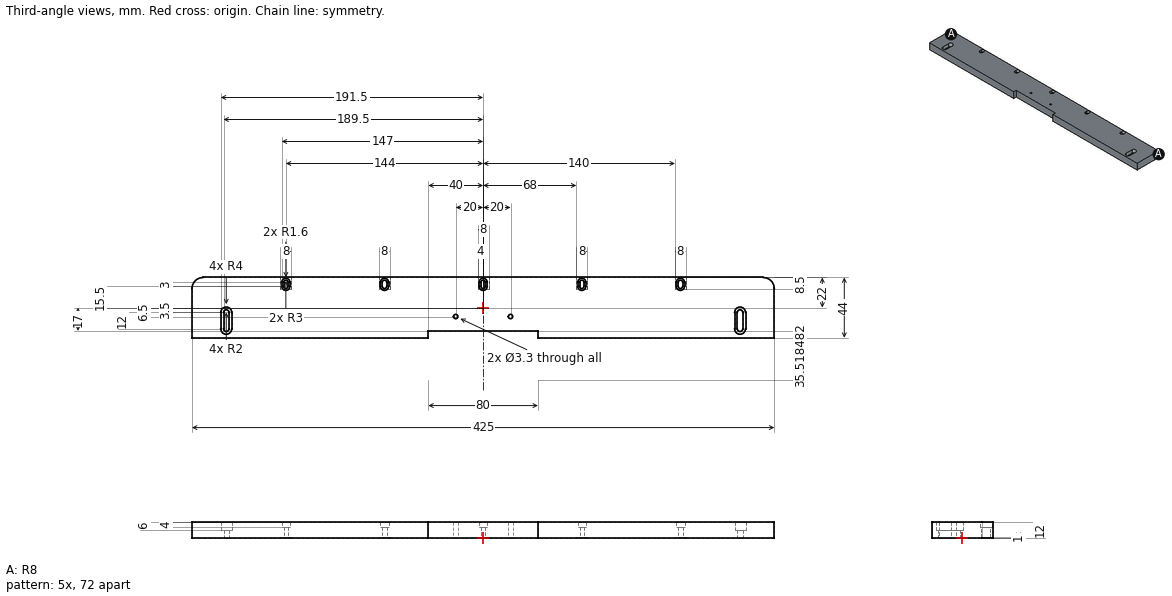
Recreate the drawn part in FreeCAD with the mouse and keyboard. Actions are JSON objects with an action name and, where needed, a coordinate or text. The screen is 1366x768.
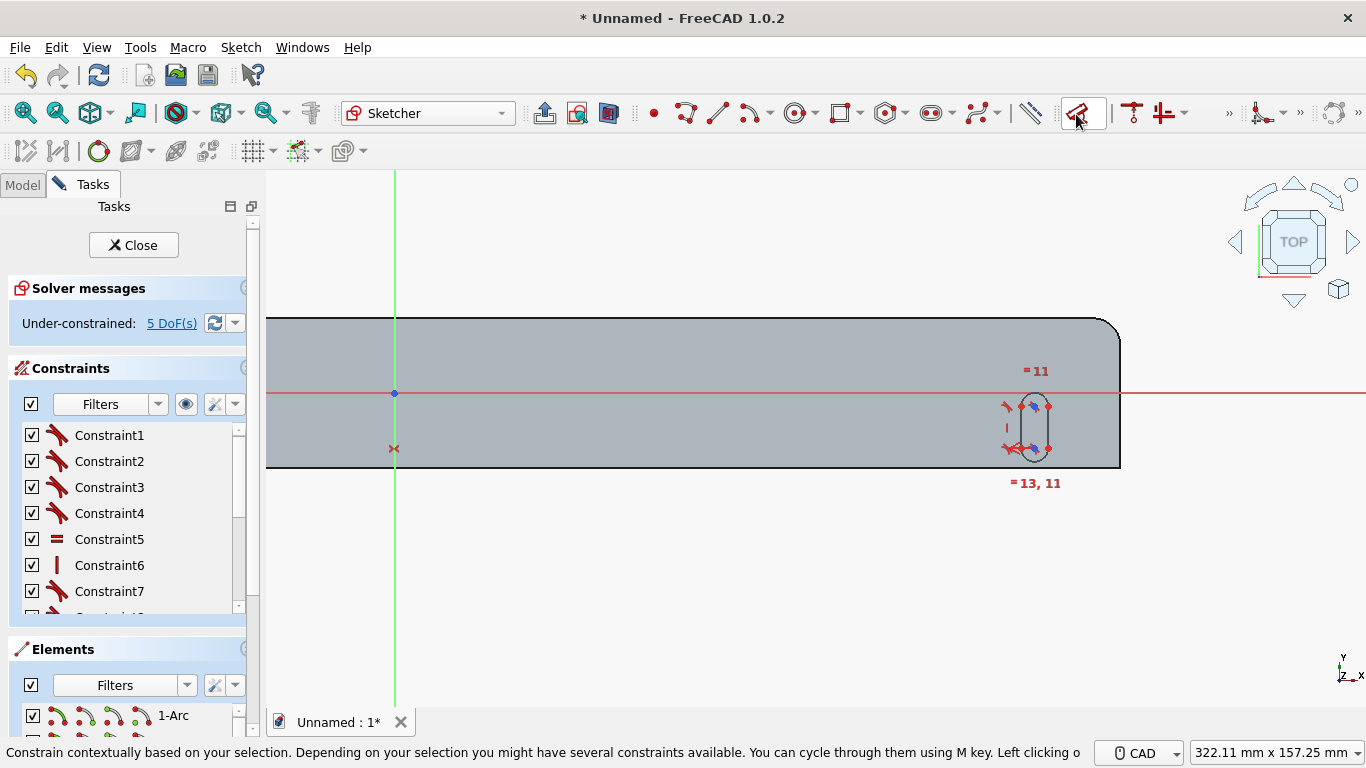
{"action": "scroll", "coordinate": [1035, 449], "scroll_direction": "down", "scroll_amount": 4}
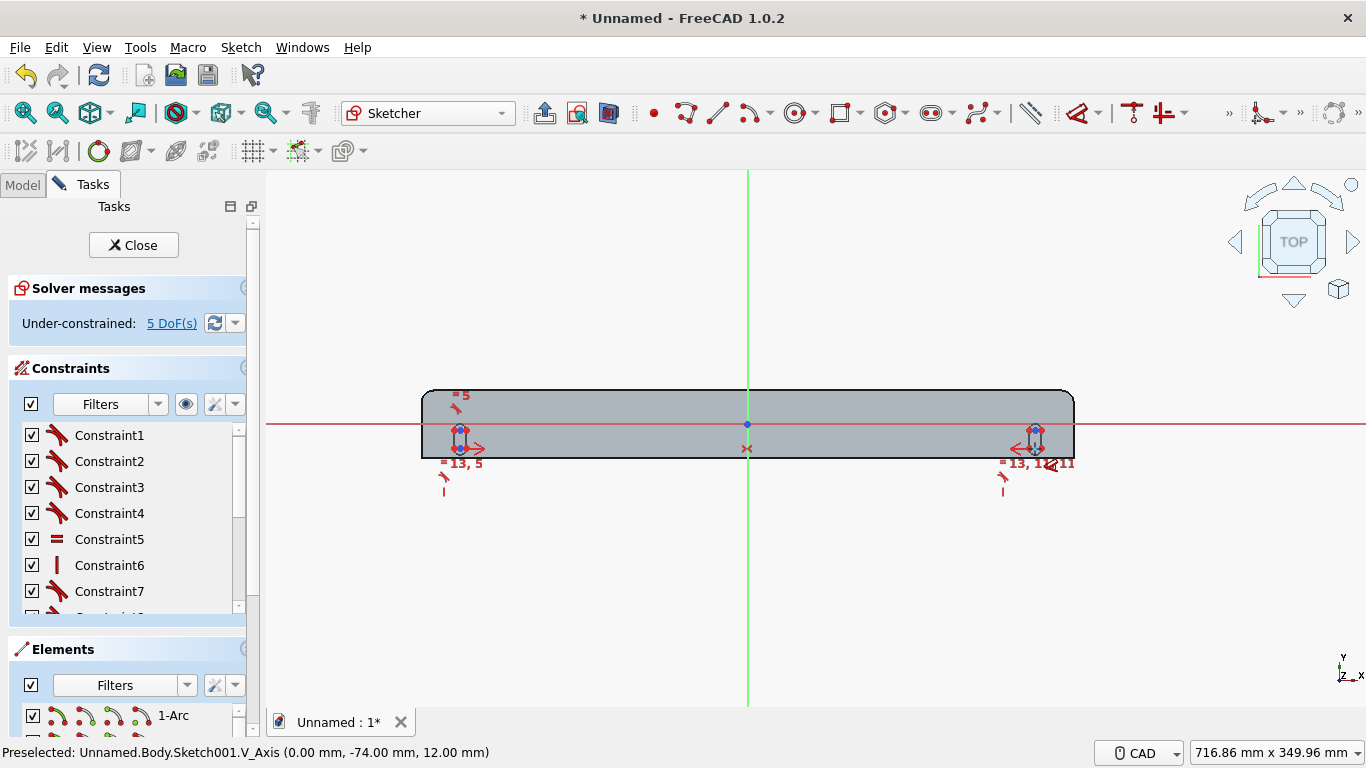
{"action": "scroll", "coordinate": [456, 454], "scroll_direction": "up", "scroll_amount": 10}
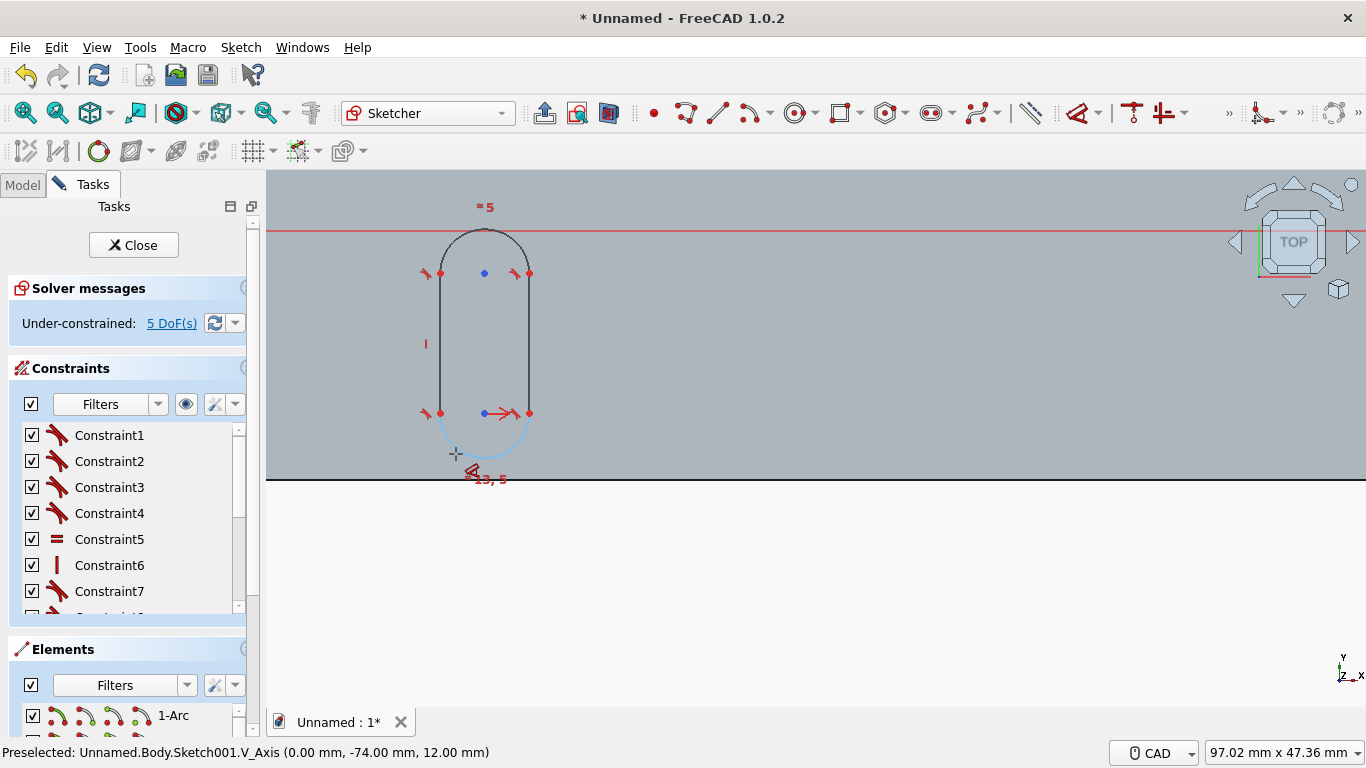
{"action": "left_click", "coordinate": [459, 450]}
{"action": "left_click", "coordinate": [441, 476]}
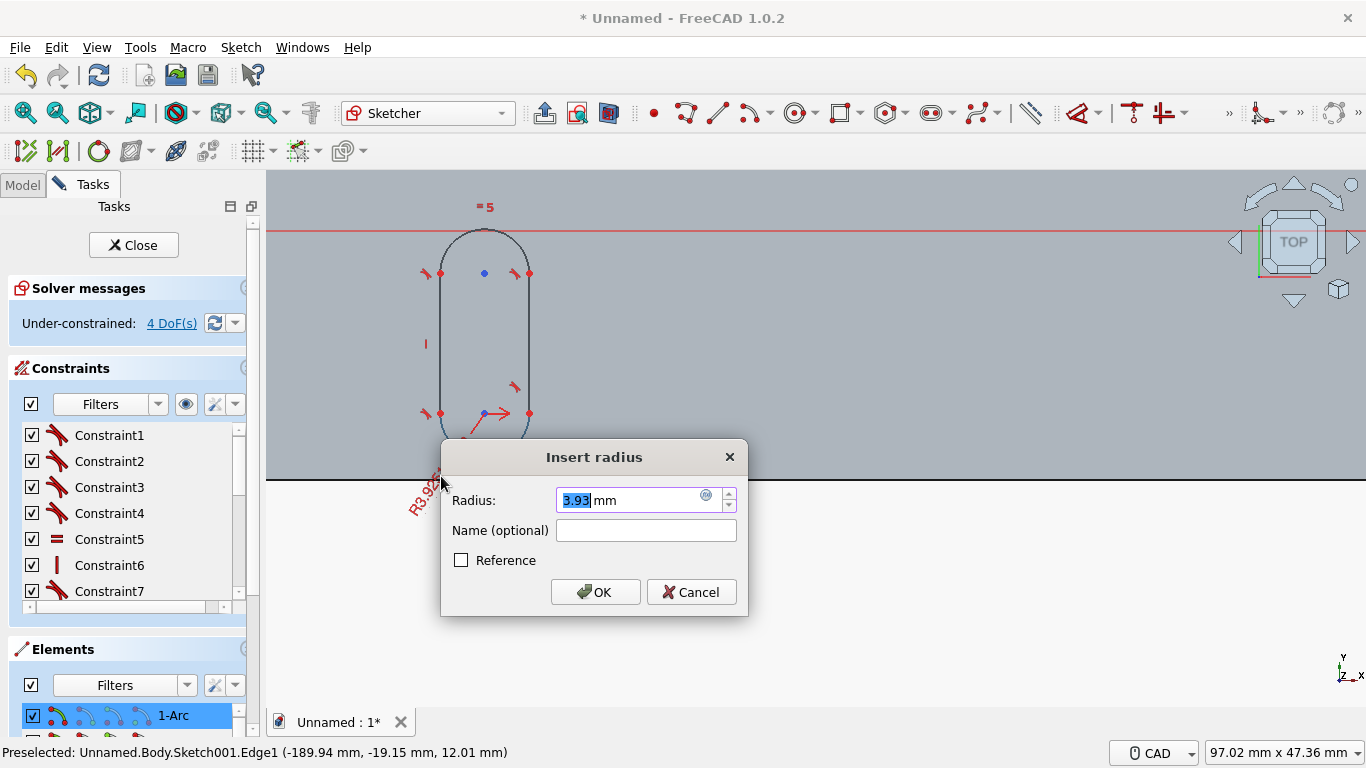
{"action": "type", "text": "4"}
{"action": "key", "text": "Return"}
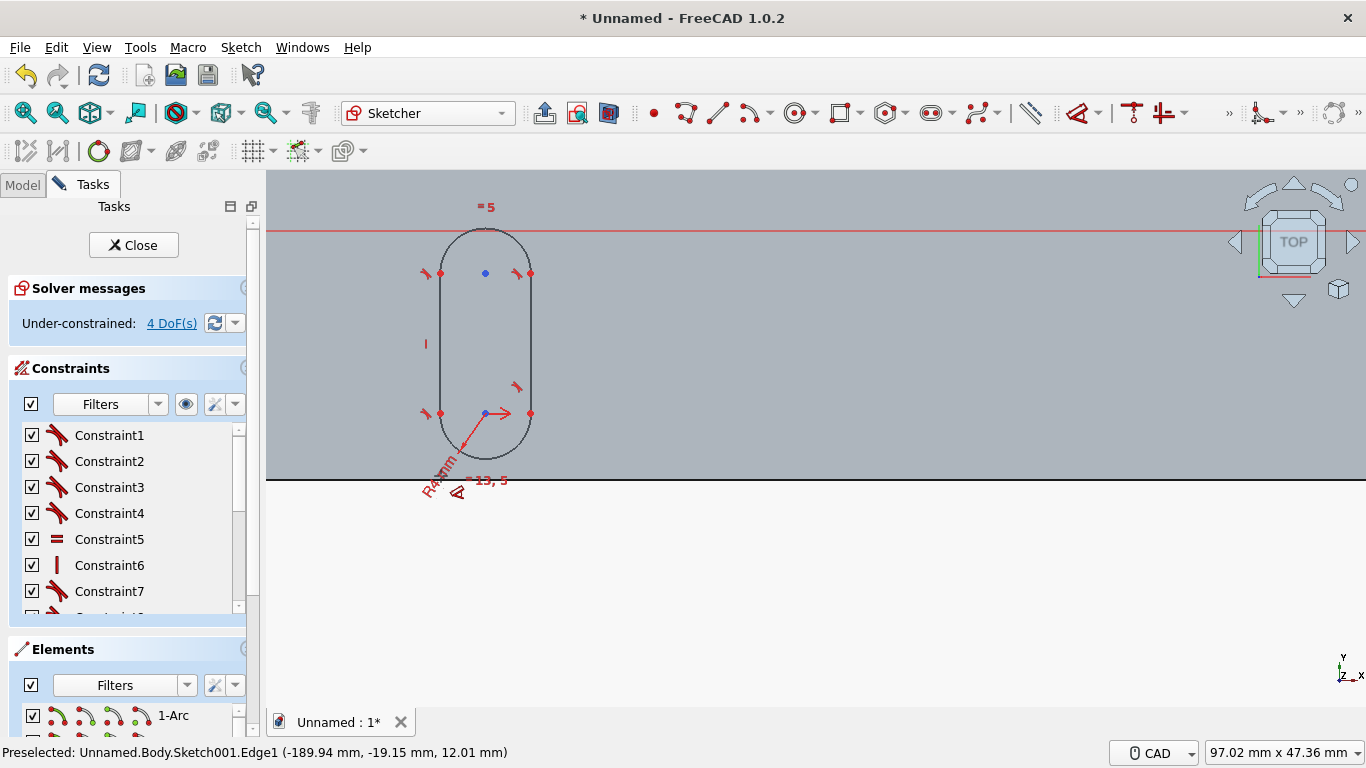
{"action": "scroll", "coordinate": [456, 454], "scroll_direction": "down", "scroll_amount": 10}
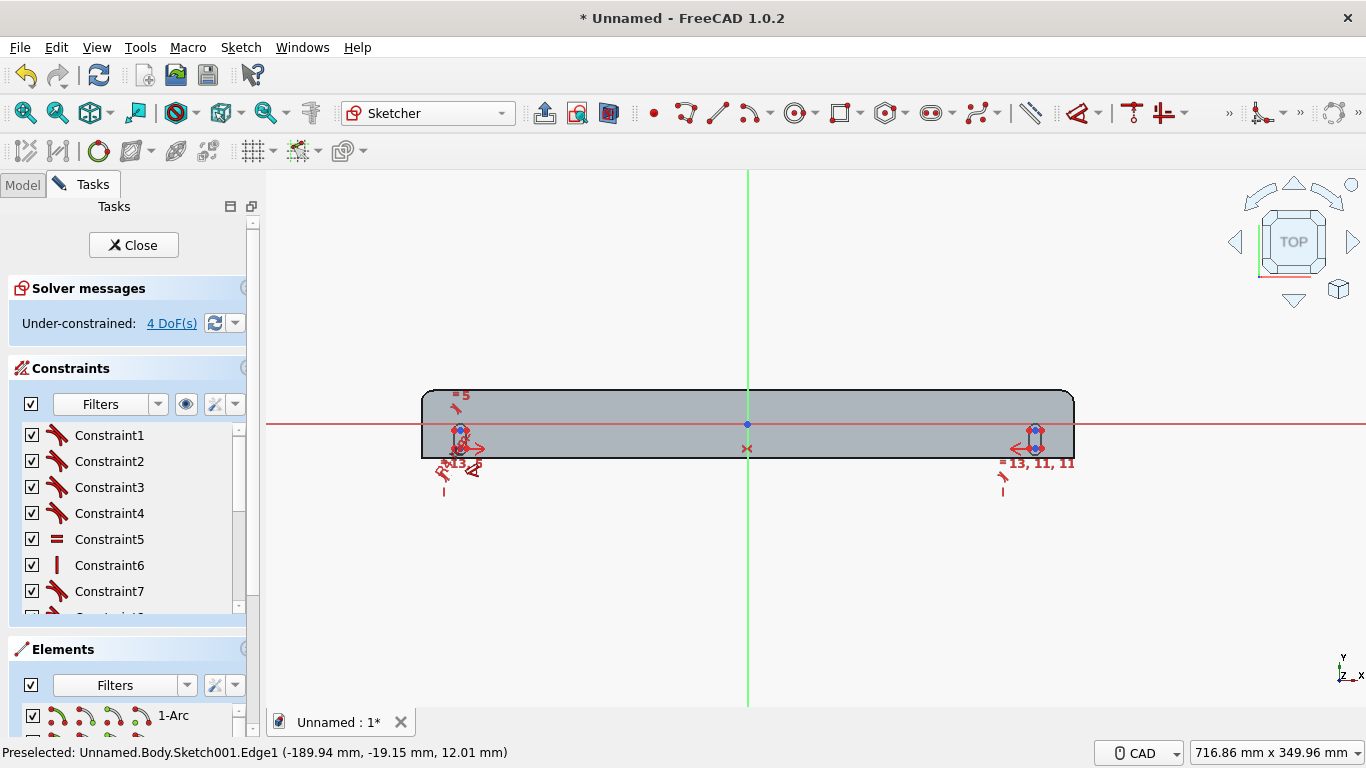
{"action": "scroll", "coordinate": [454, 443], "scroll_direction": "up", "scroll_amount": 5}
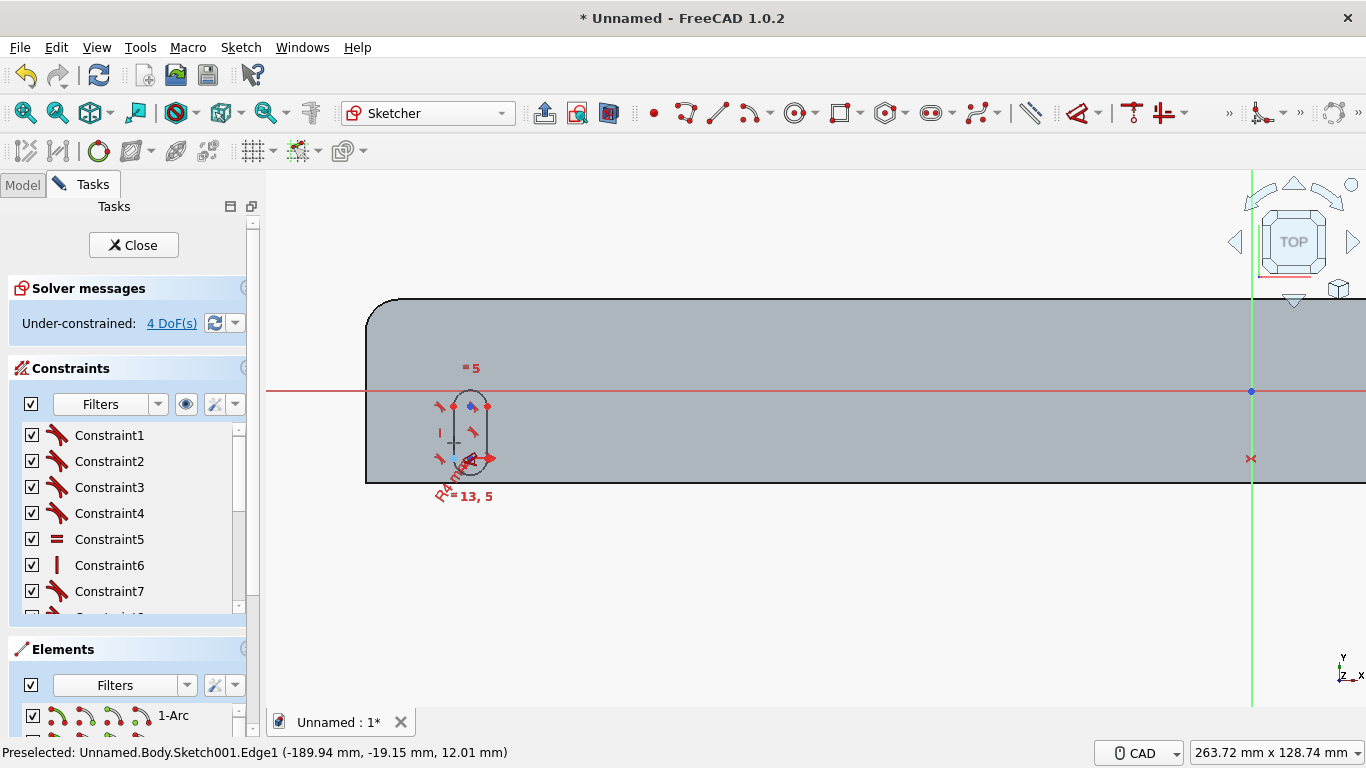
{"action": "left_click", "coordinate": [454, 443]}
{"action": "left_click", "coordinate": [420, 433]}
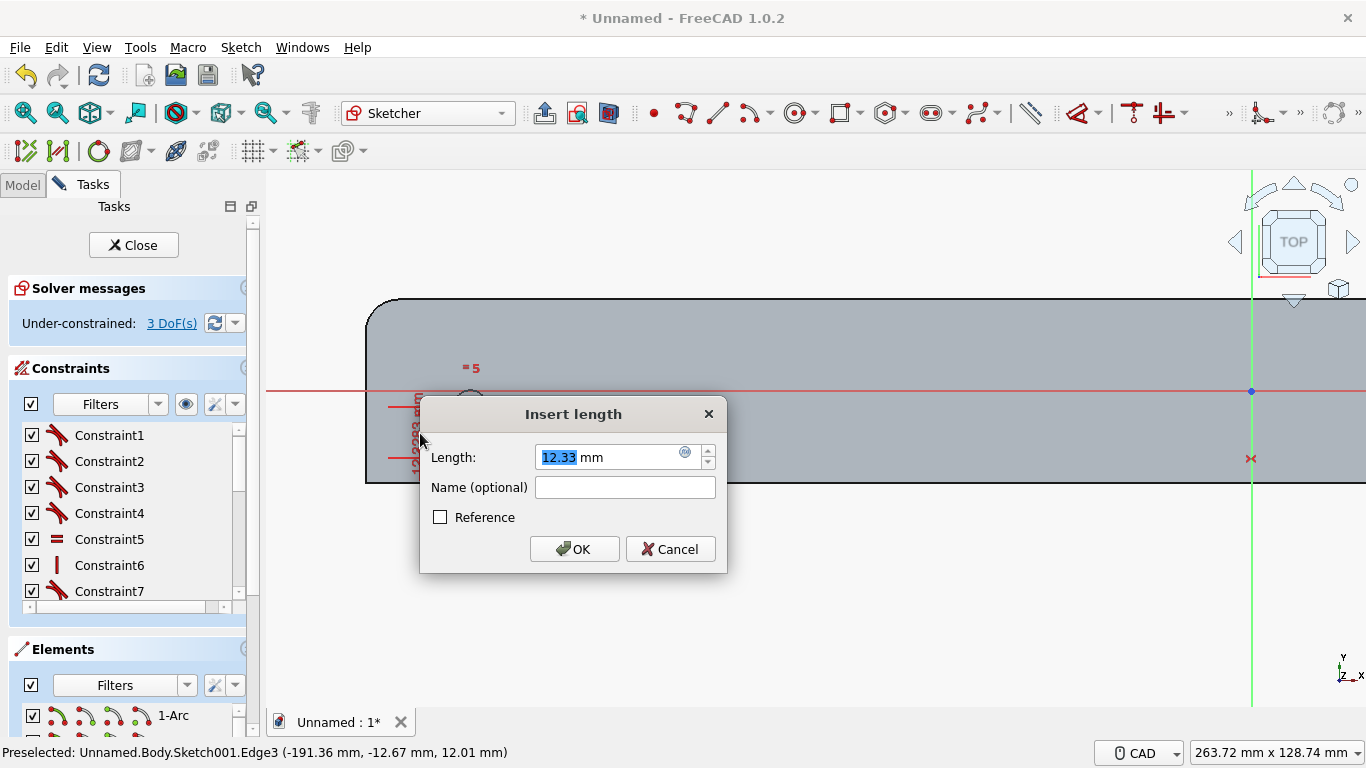
{"action": "type", "text": "12"}
{"action": "key", "text": "Return"}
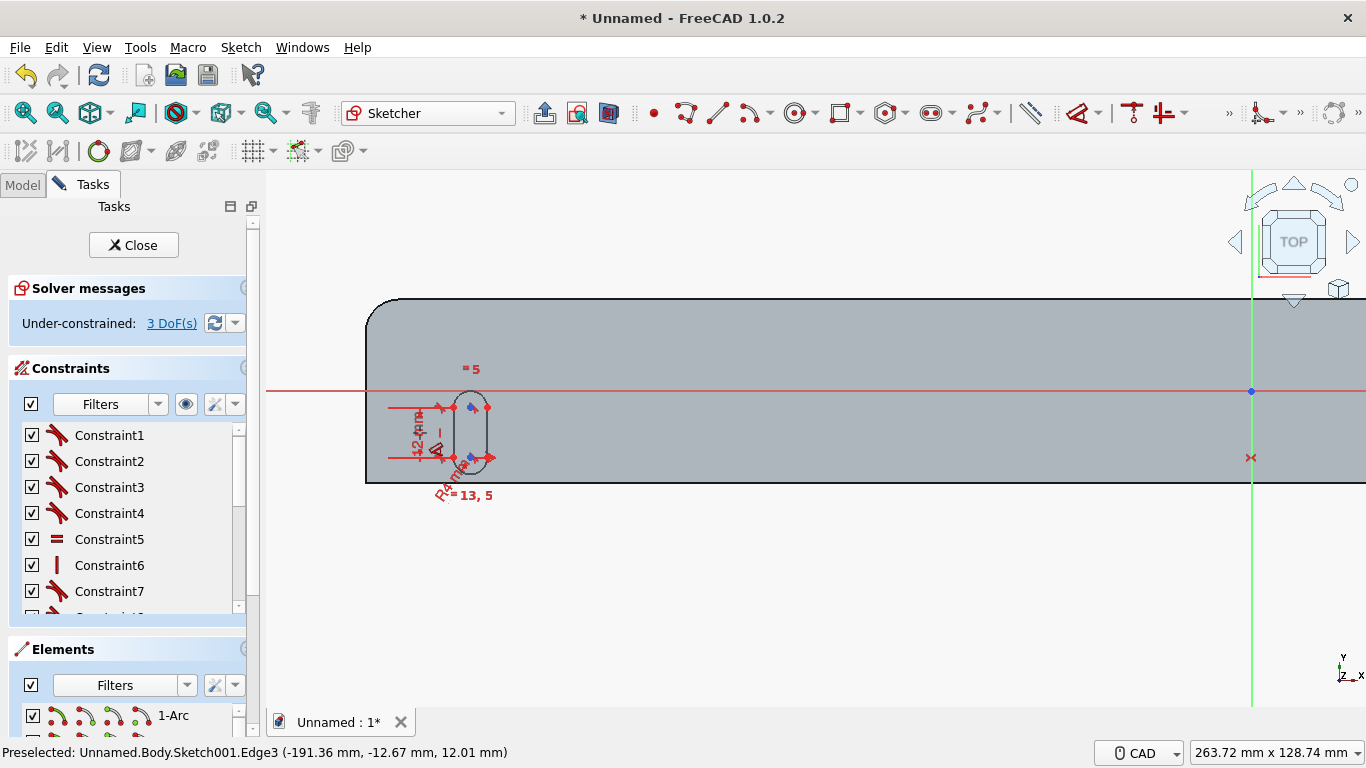
{"action": "scroll", "coordinate": [454, 443], "scroll_direction": "down", "scroll_amount": 5}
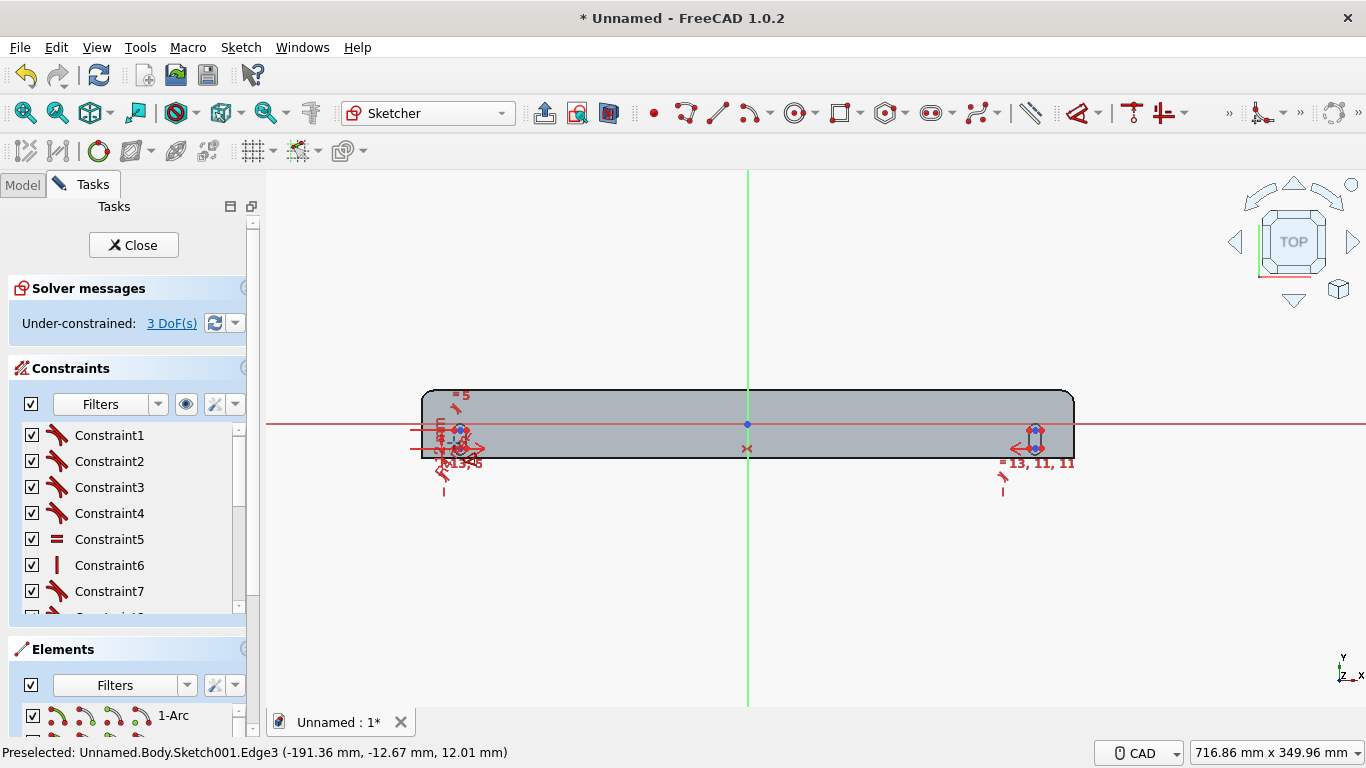
{"action": "scroll", "coordinate": [1029, 443], "scroll_direction": "up", "scroll_amount": 5}